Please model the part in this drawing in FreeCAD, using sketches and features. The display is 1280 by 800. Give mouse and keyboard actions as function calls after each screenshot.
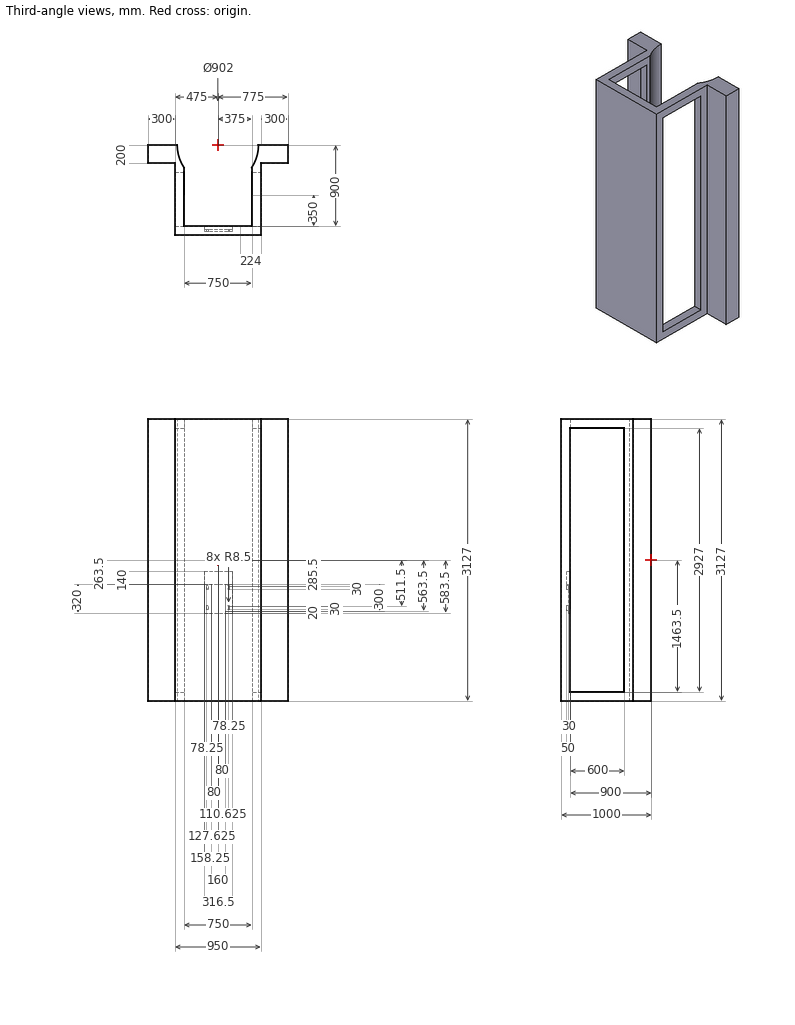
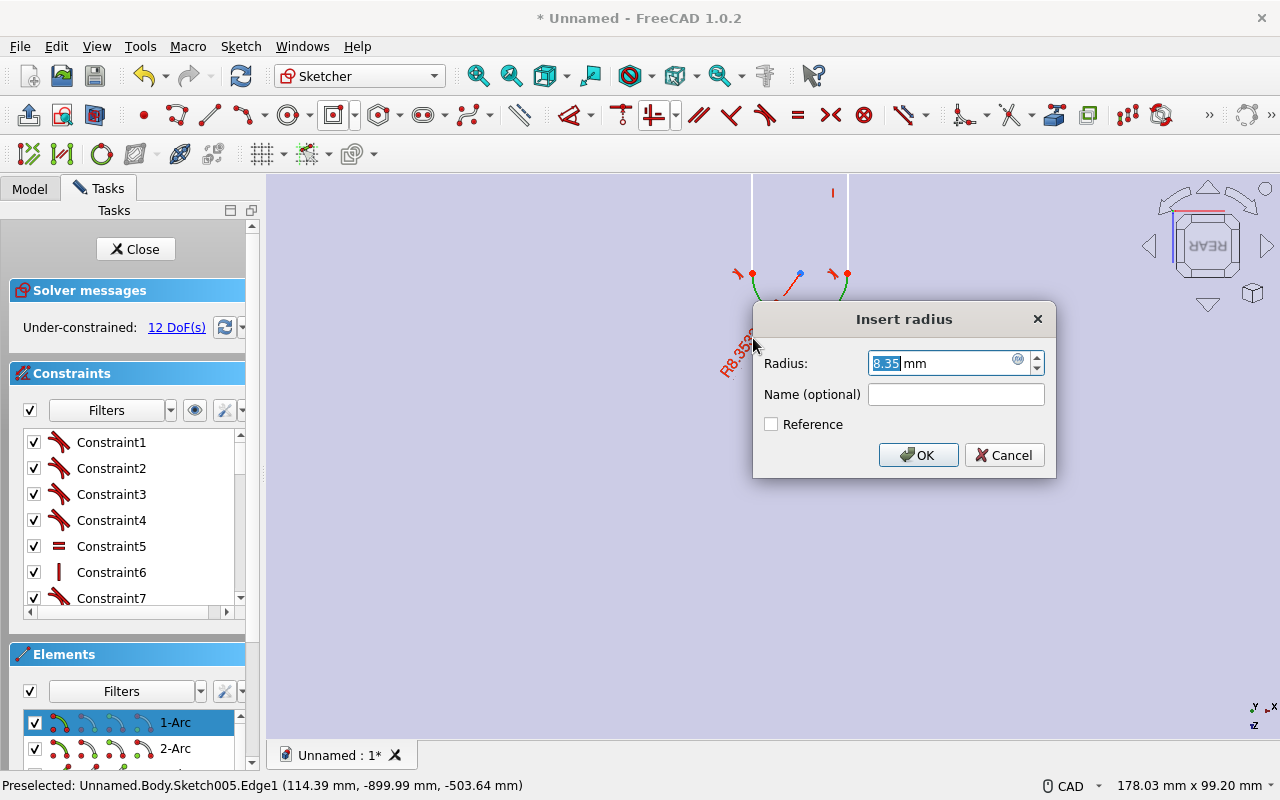
text(8.5)
key(Return)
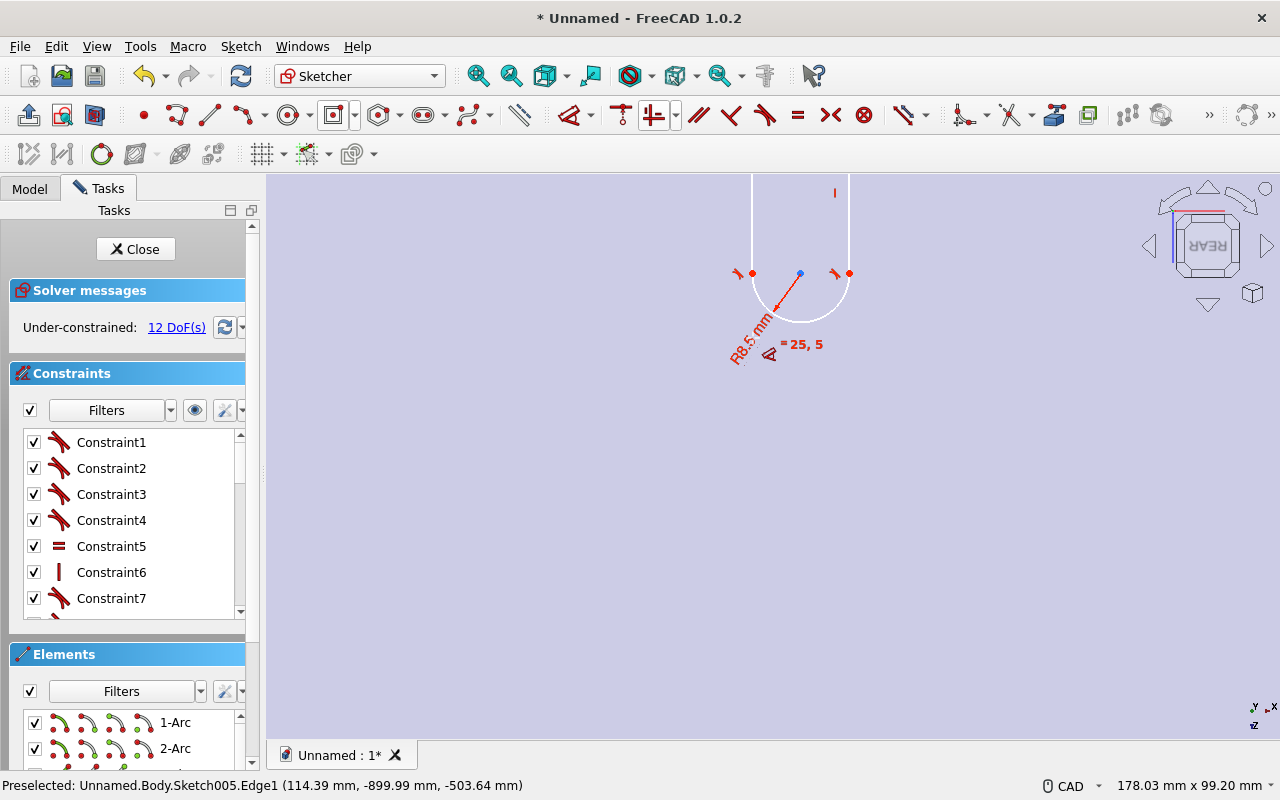
scroll(777, 312, down, 11)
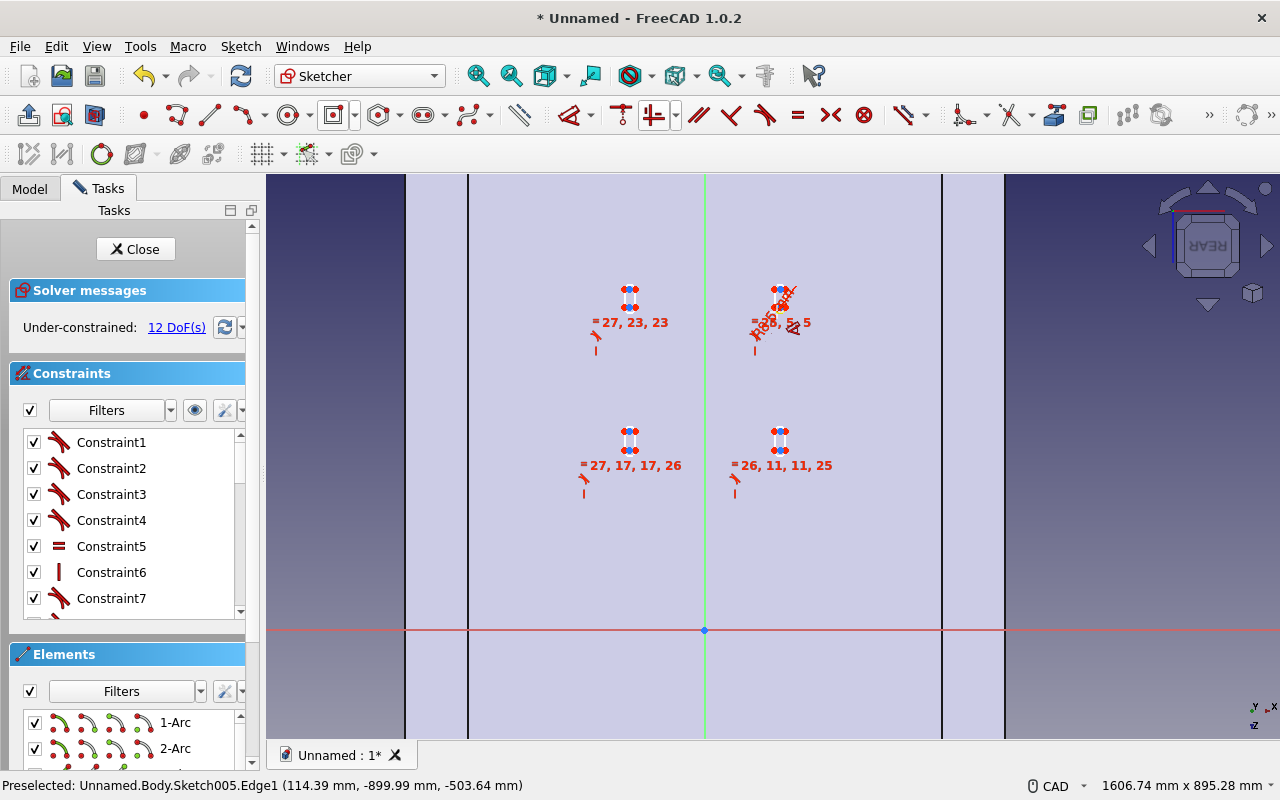
scroll(775, 303, up, 5)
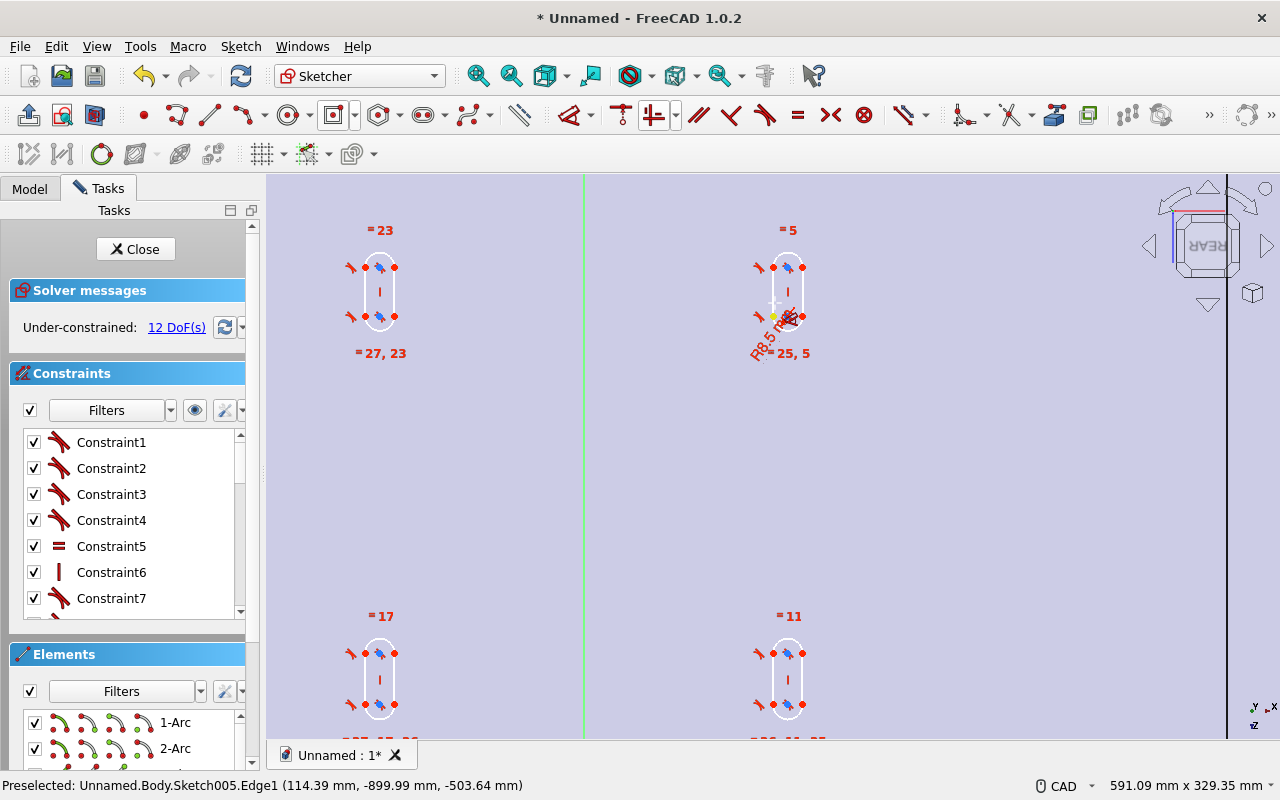
click(773, 302)
click(739, 292)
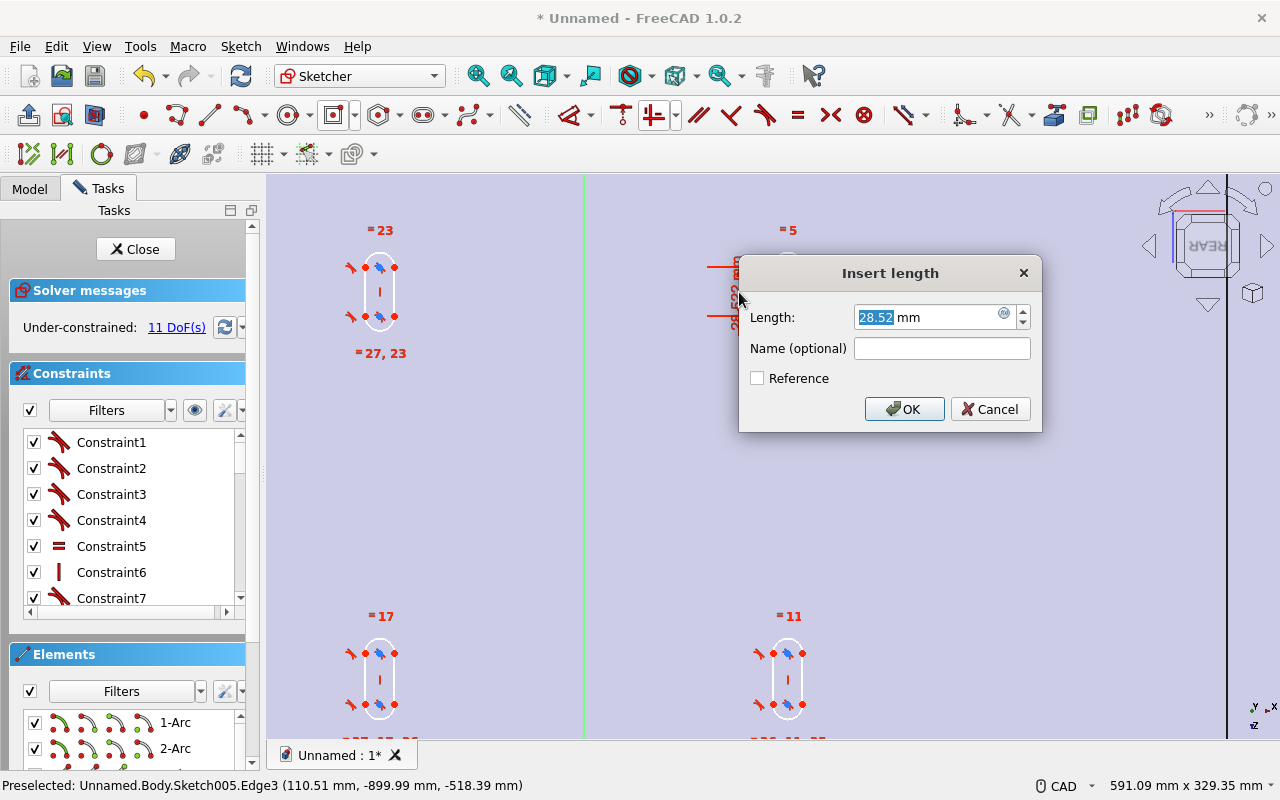
text(30)
key(Return)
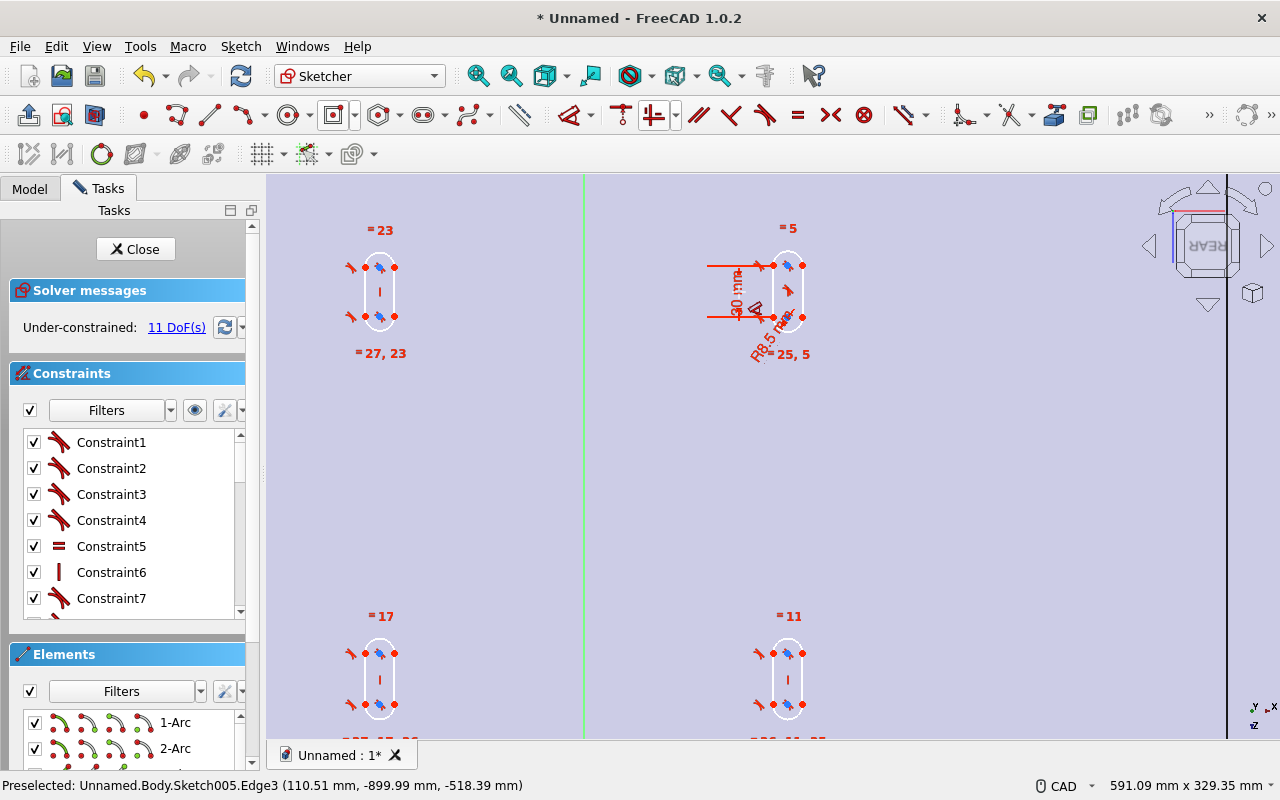
click(773, 689)
click(739, 679)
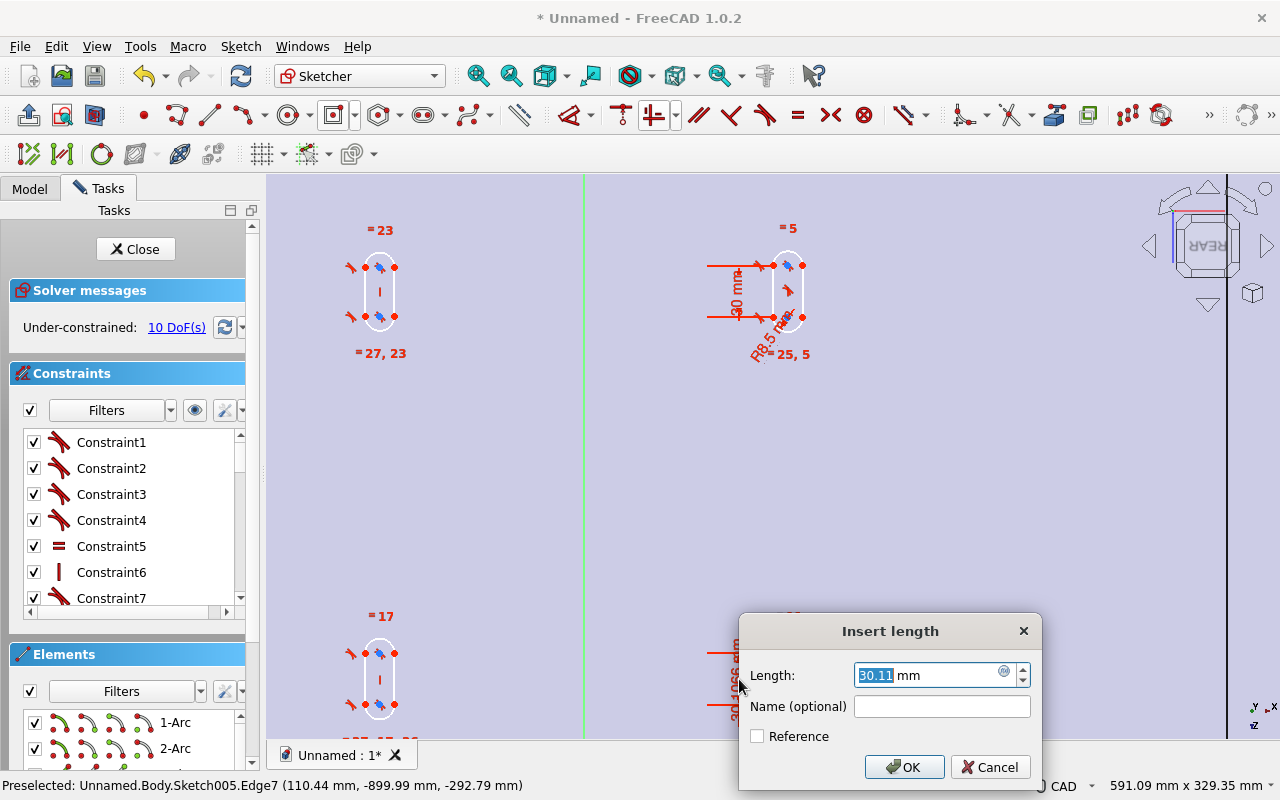
text(30)
key(Return)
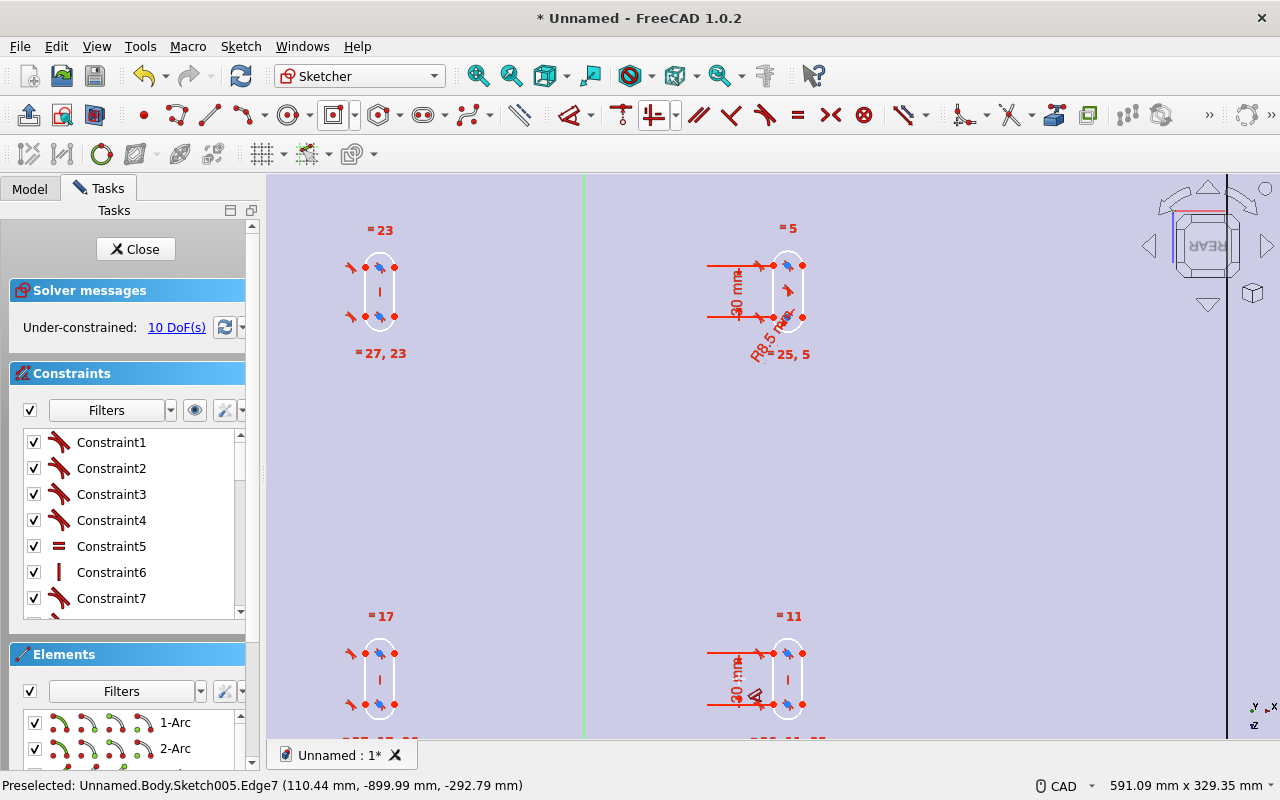
click(365, 689)
click(331, 679)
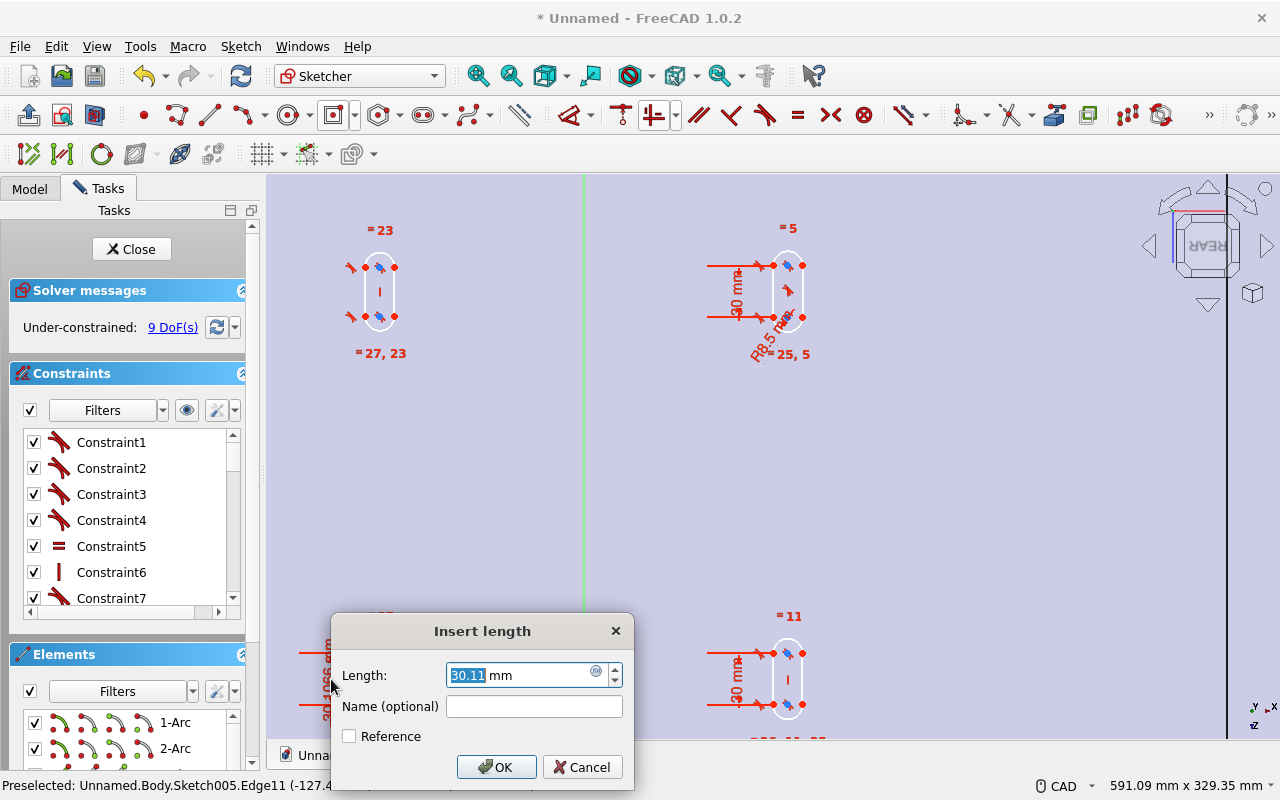
text(30)
key(Return)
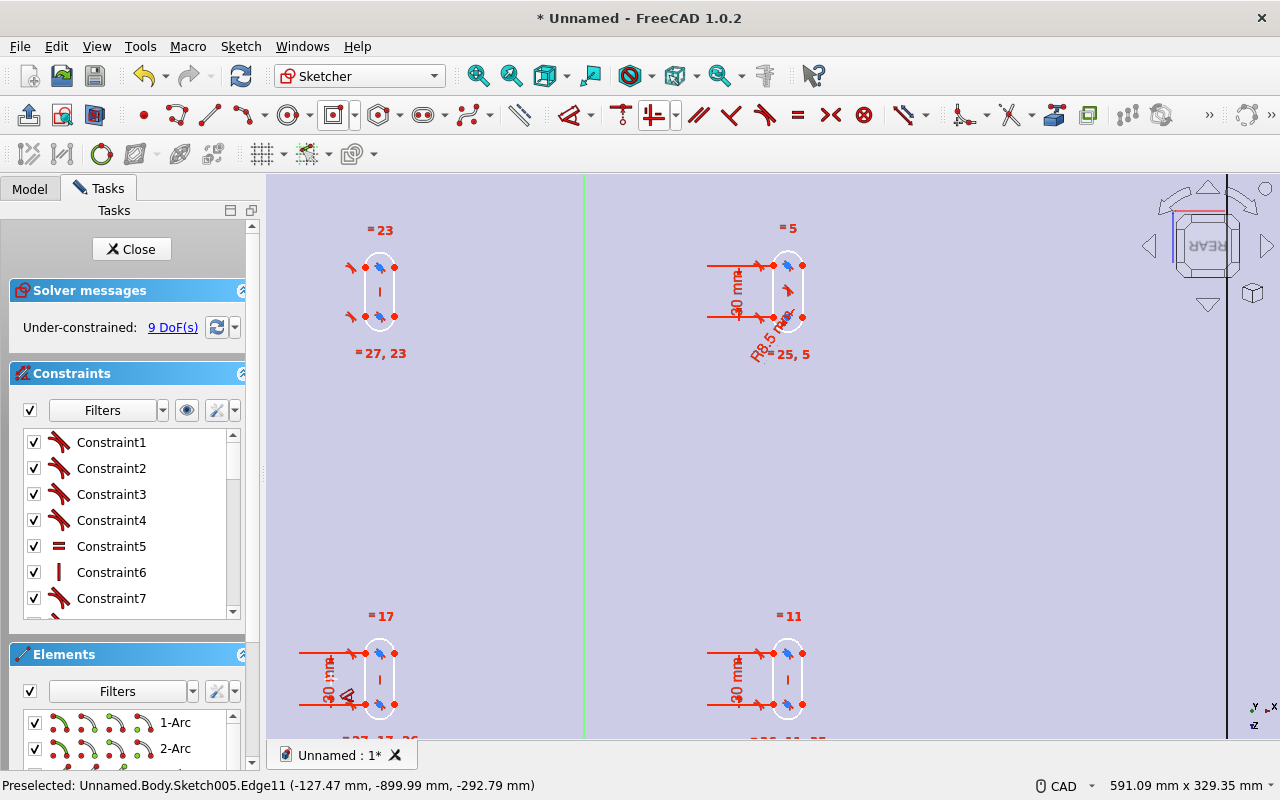
click(365, 302)
click(331, 292)